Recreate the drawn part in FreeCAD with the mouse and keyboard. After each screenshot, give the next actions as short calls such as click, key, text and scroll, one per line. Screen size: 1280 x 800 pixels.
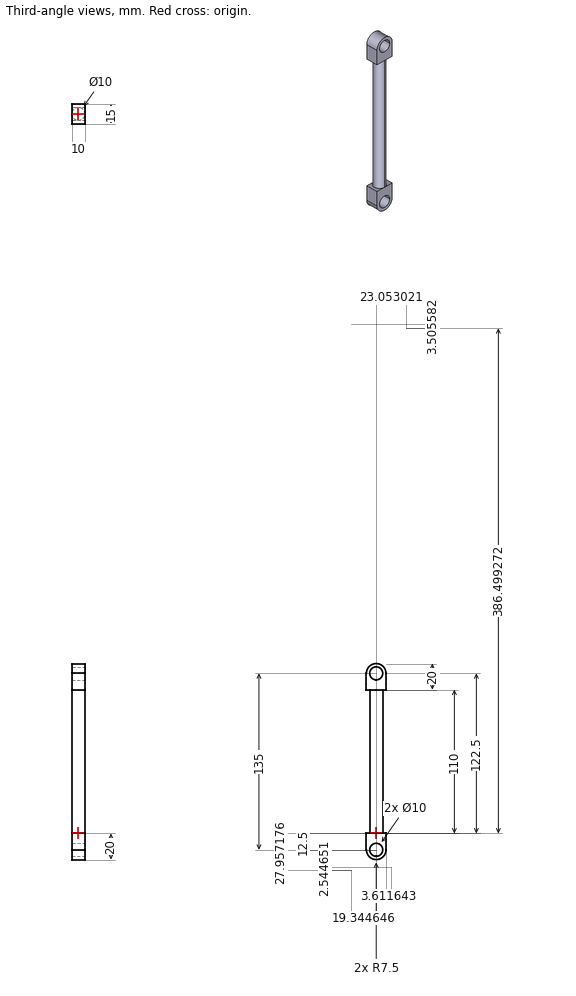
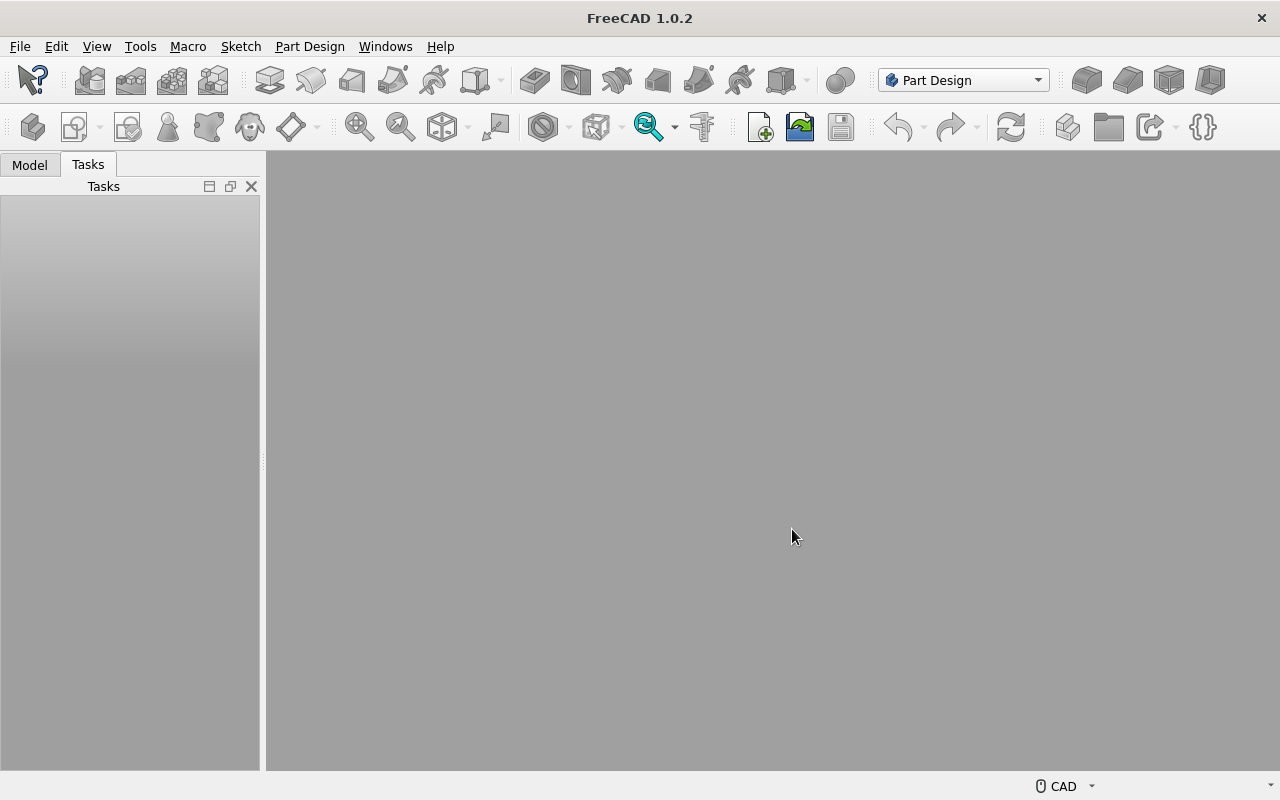
click(759, 128)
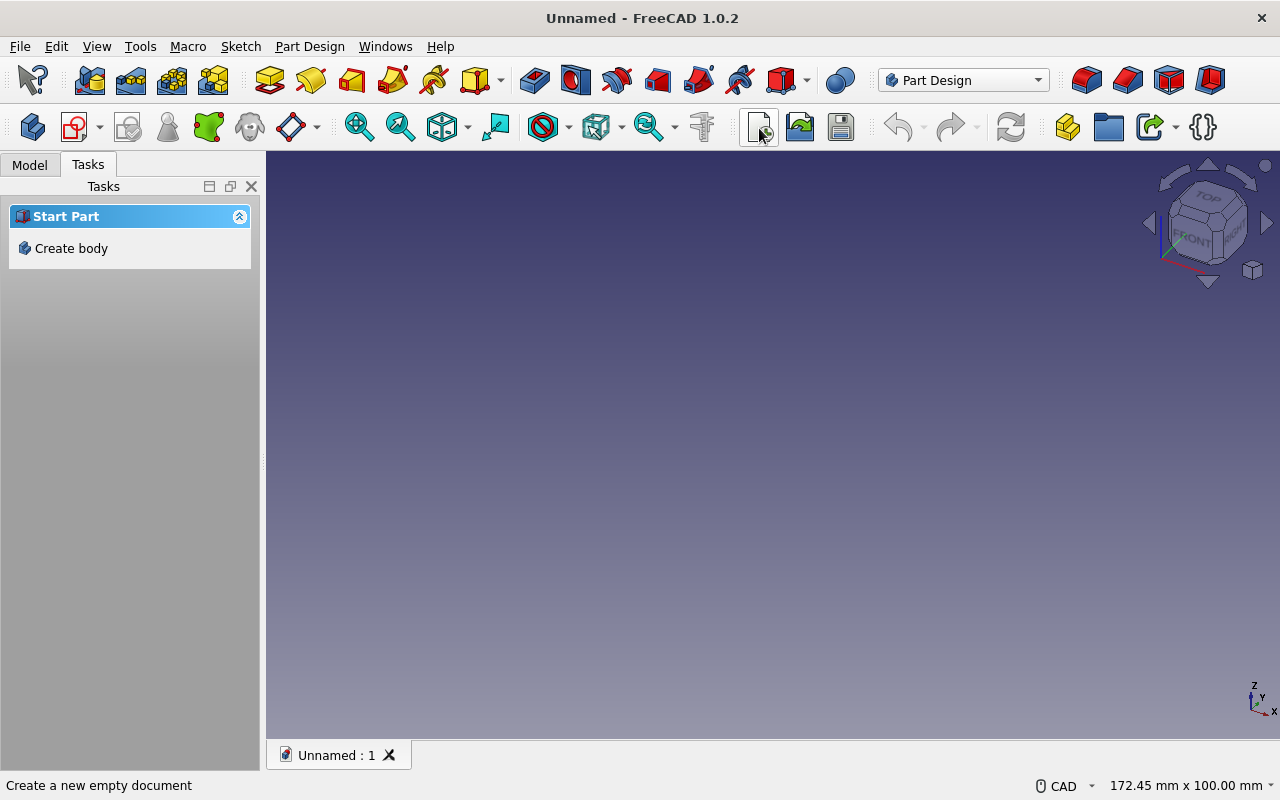
click(74, 128)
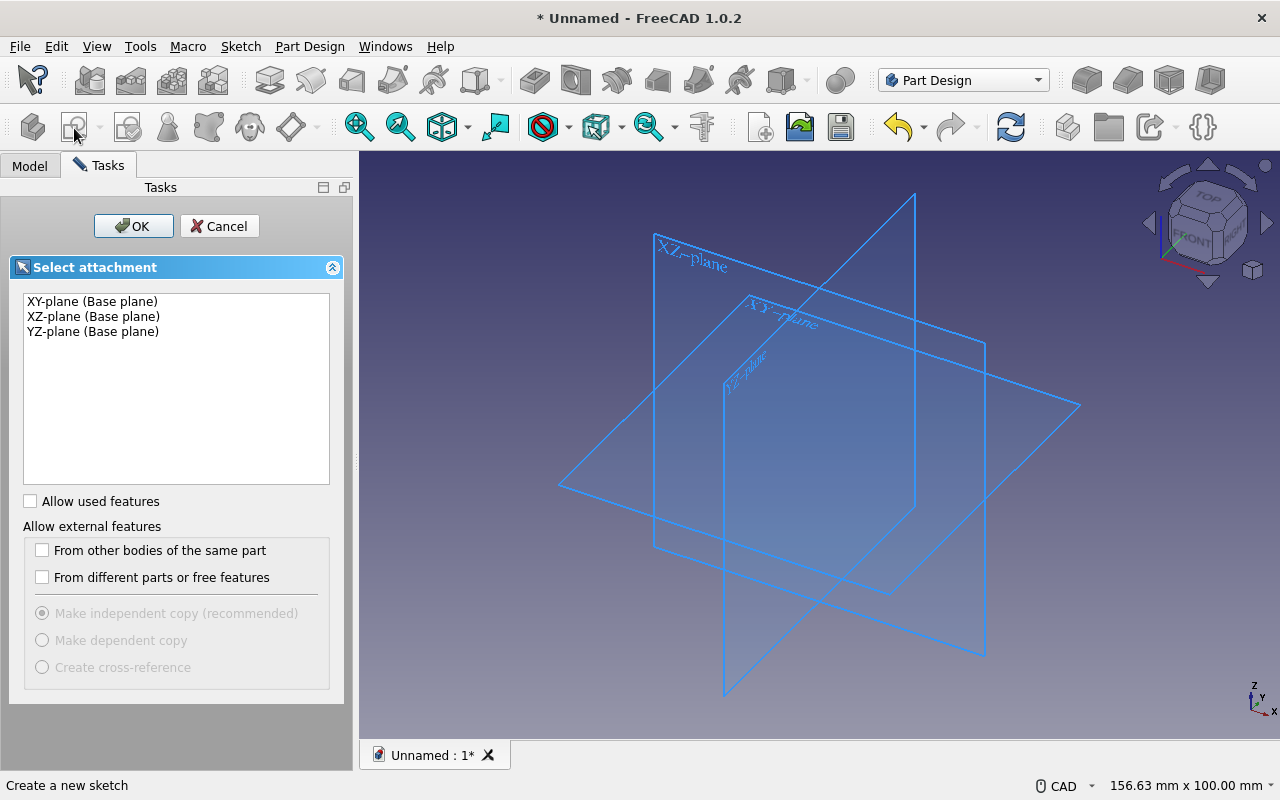
click(84, 302)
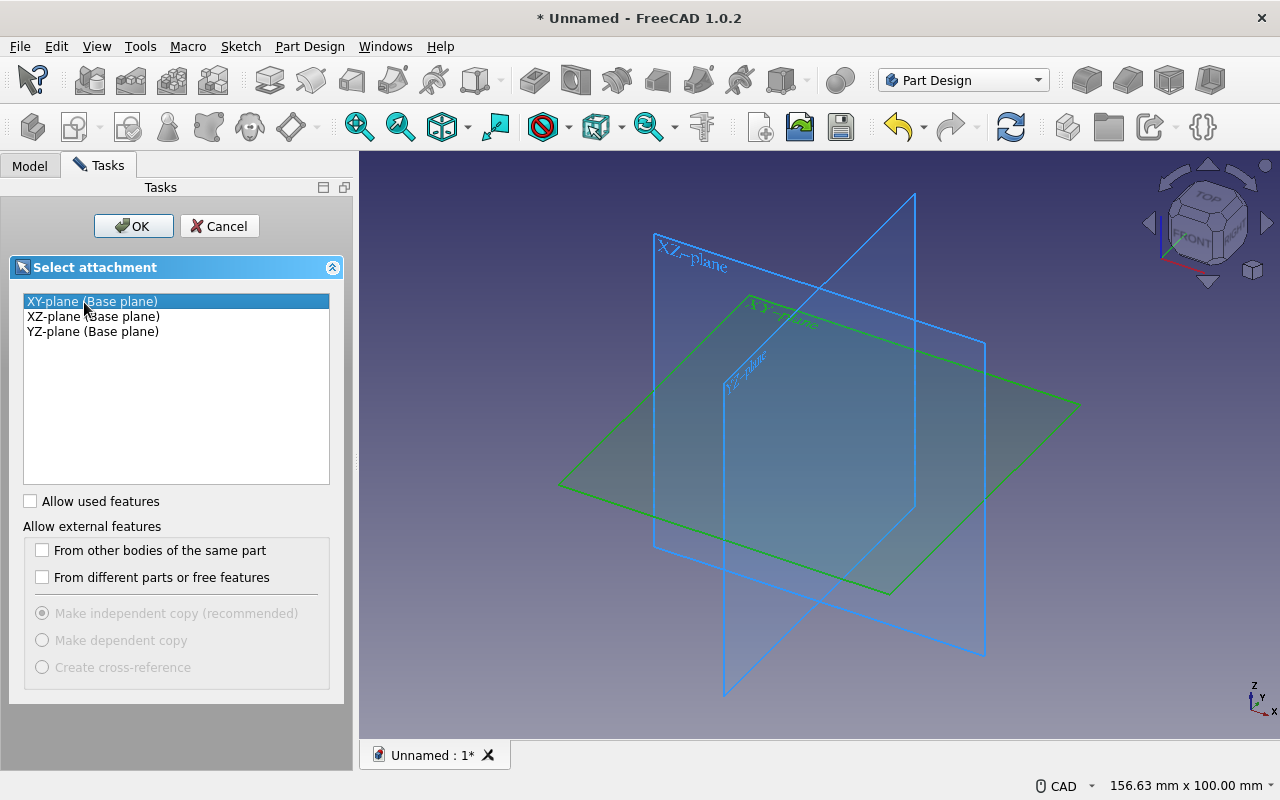
click(134, 226)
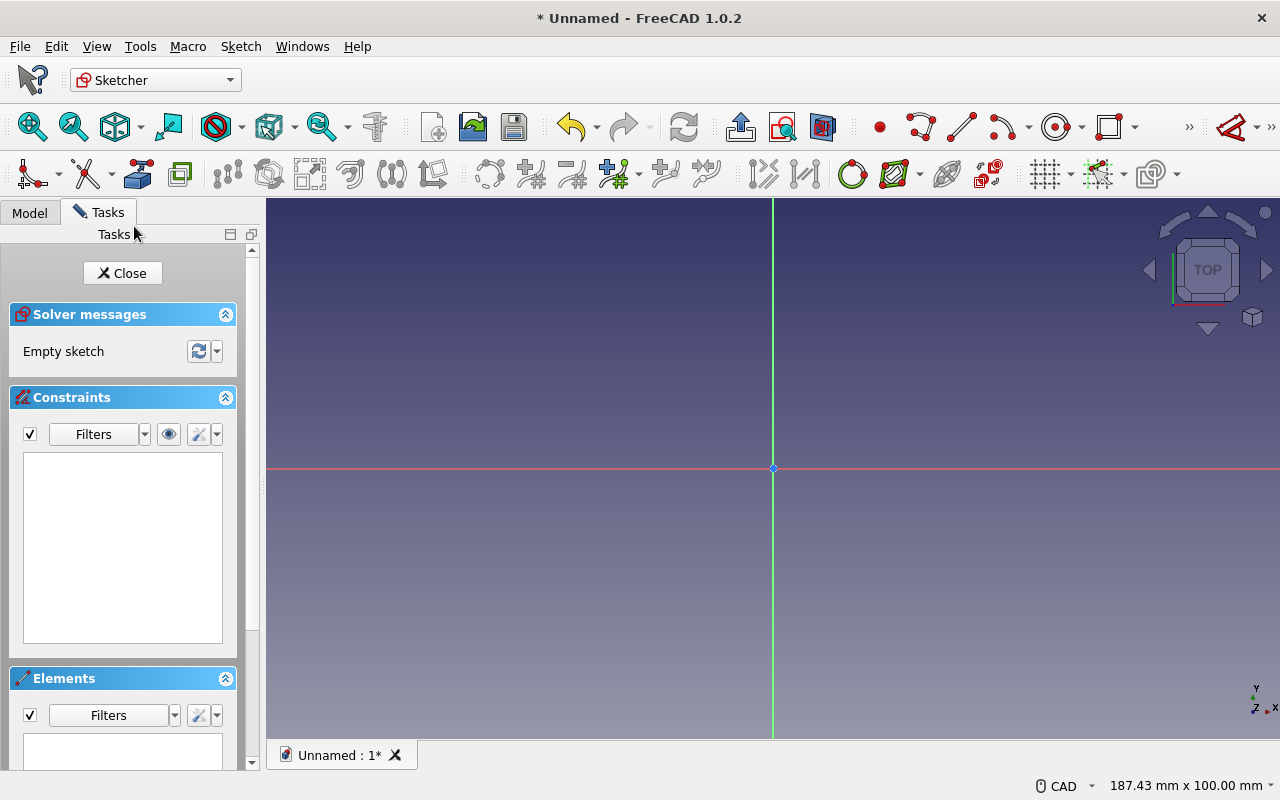
scroll(787, 468, up, 9)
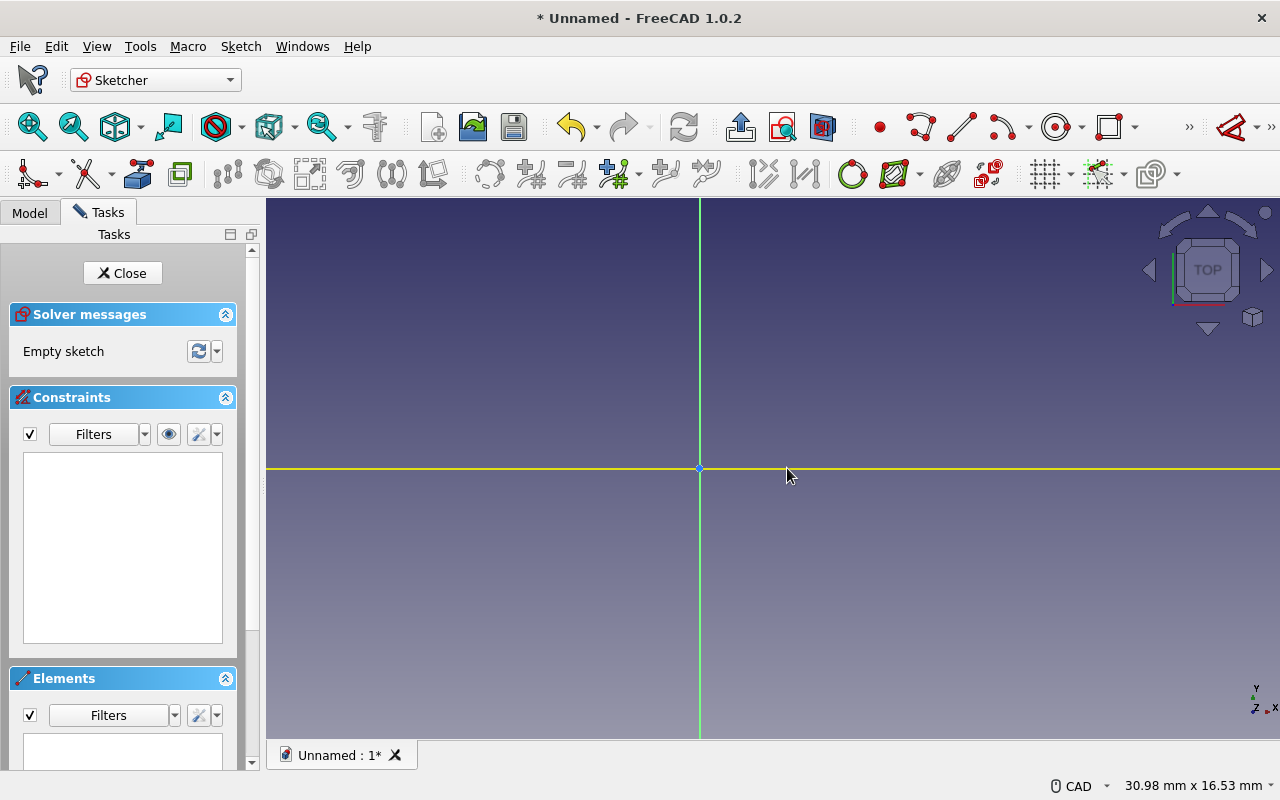
click(1056, 128)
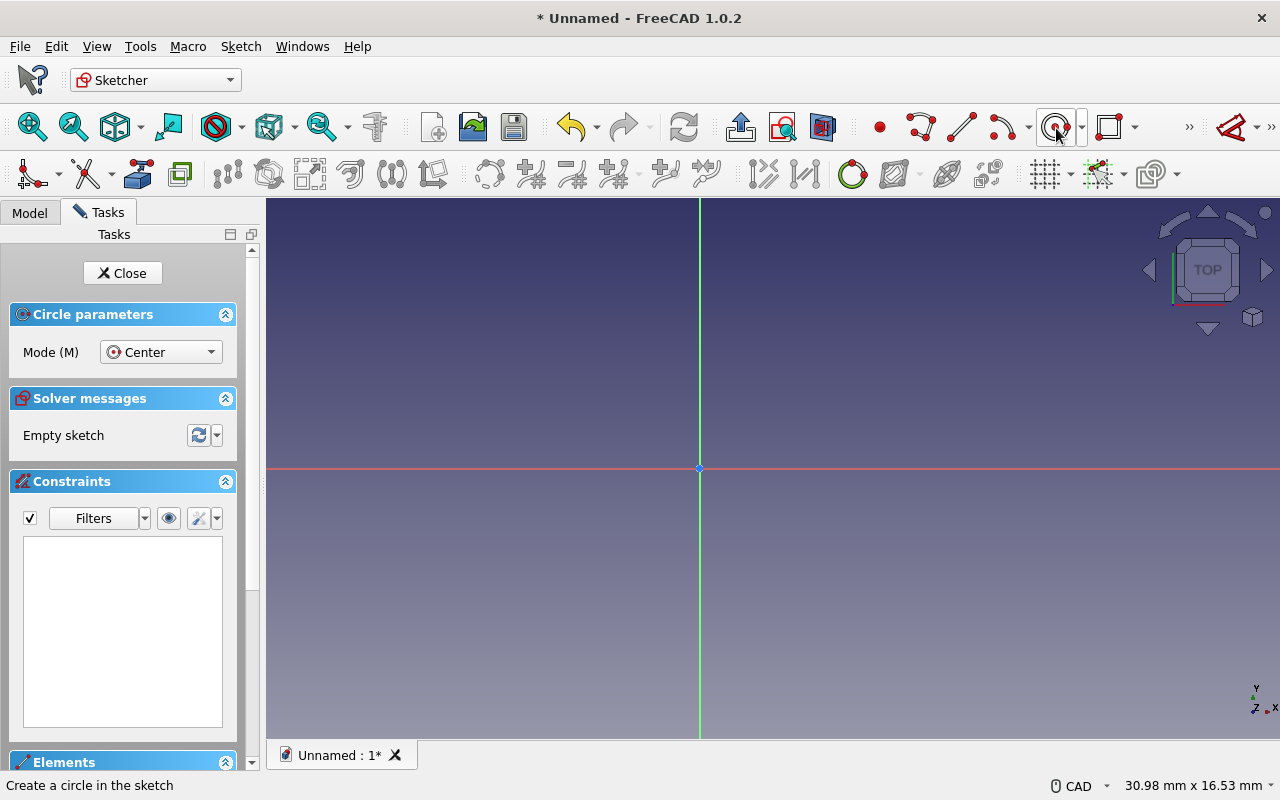
click(700, 468)
move(815, 353)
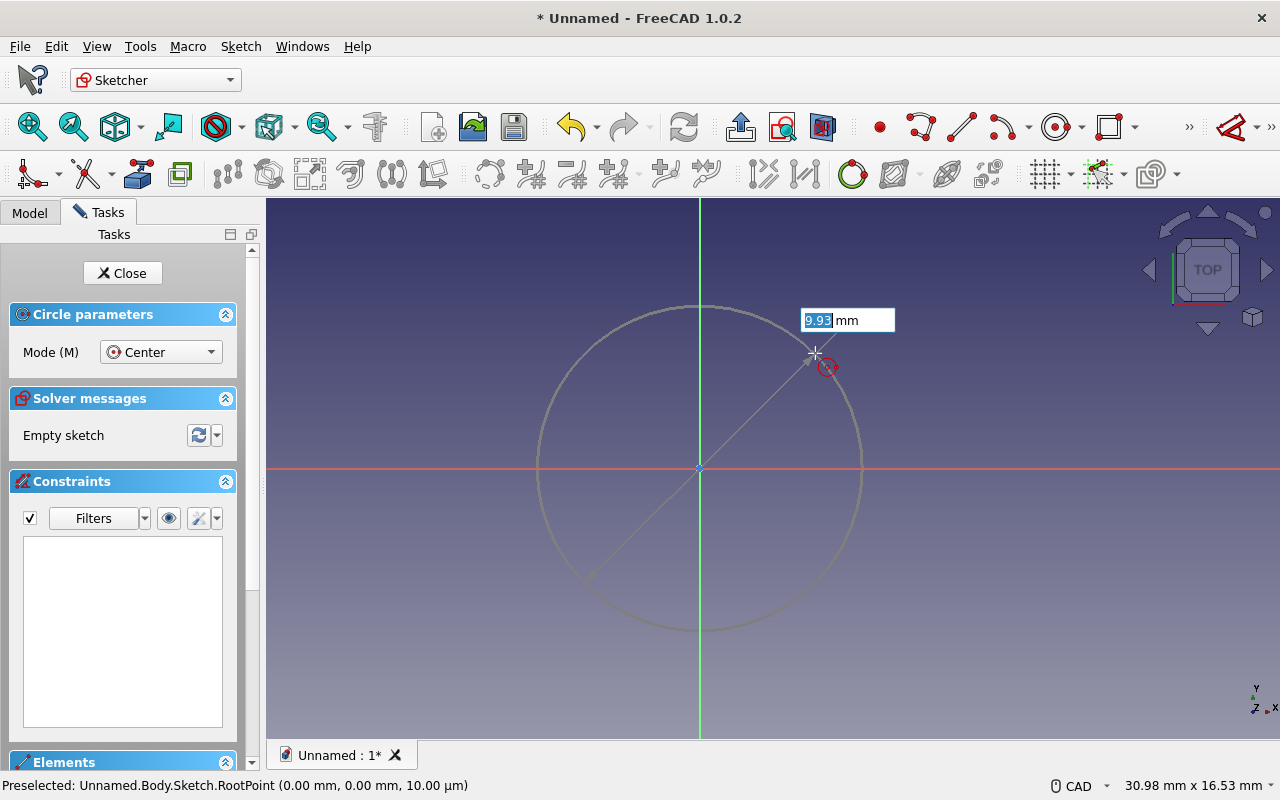
text(10)
key(Return)
key(Escape)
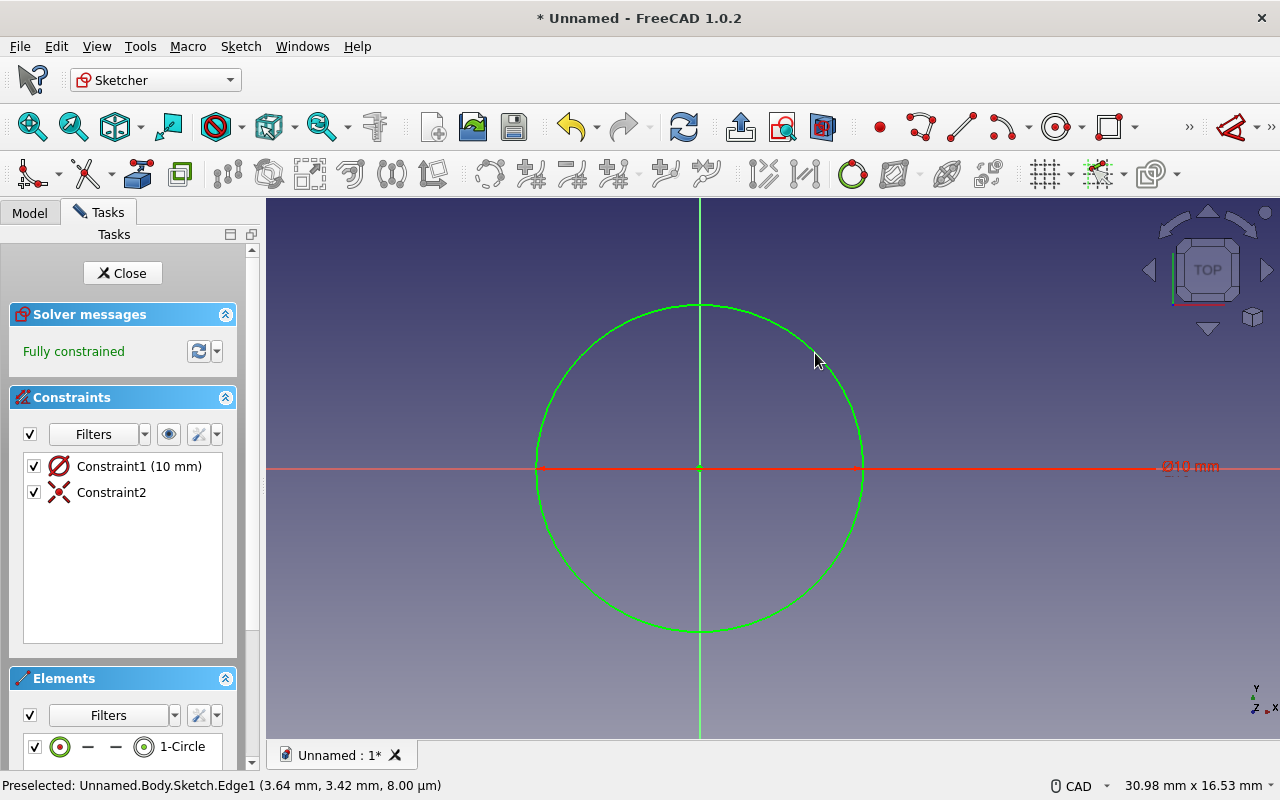
click(123, 273)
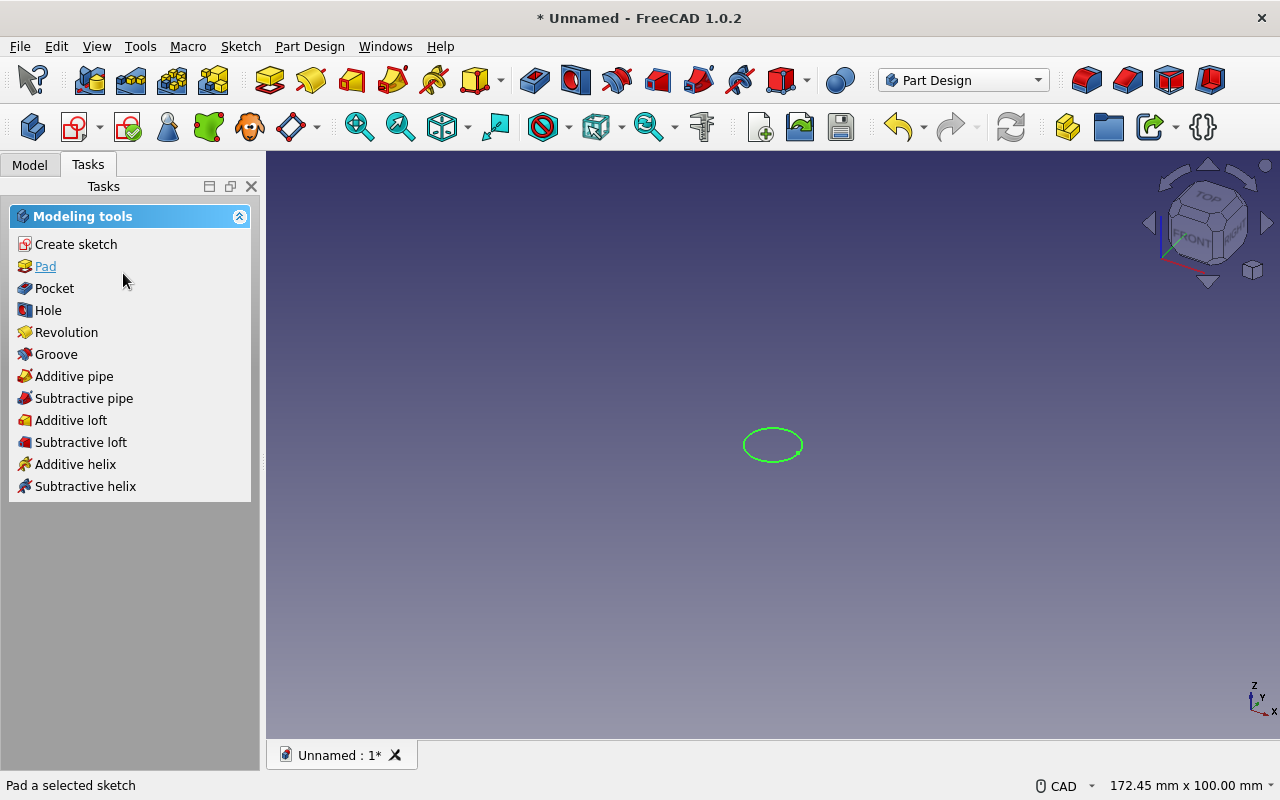
click(270, 80)